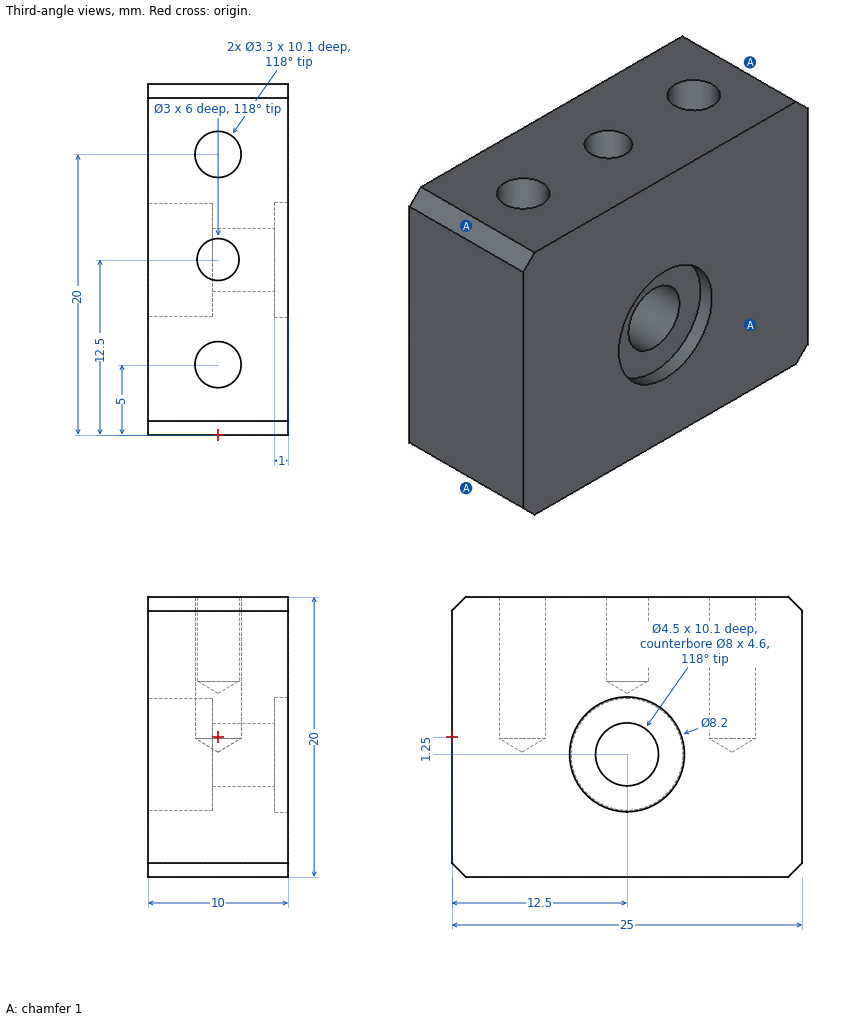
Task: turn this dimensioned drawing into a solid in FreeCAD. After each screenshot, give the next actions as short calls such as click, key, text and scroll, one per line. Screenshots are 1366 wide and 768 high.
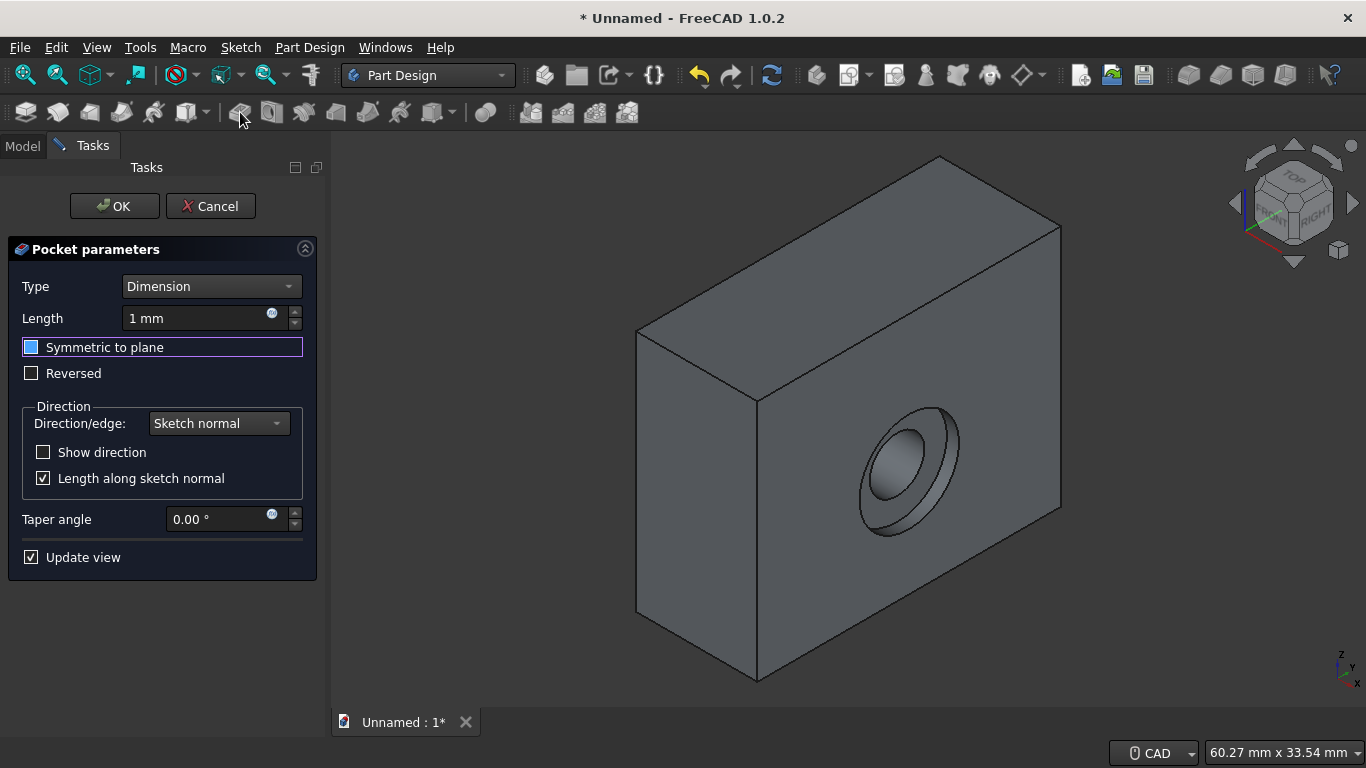
click(115, 206)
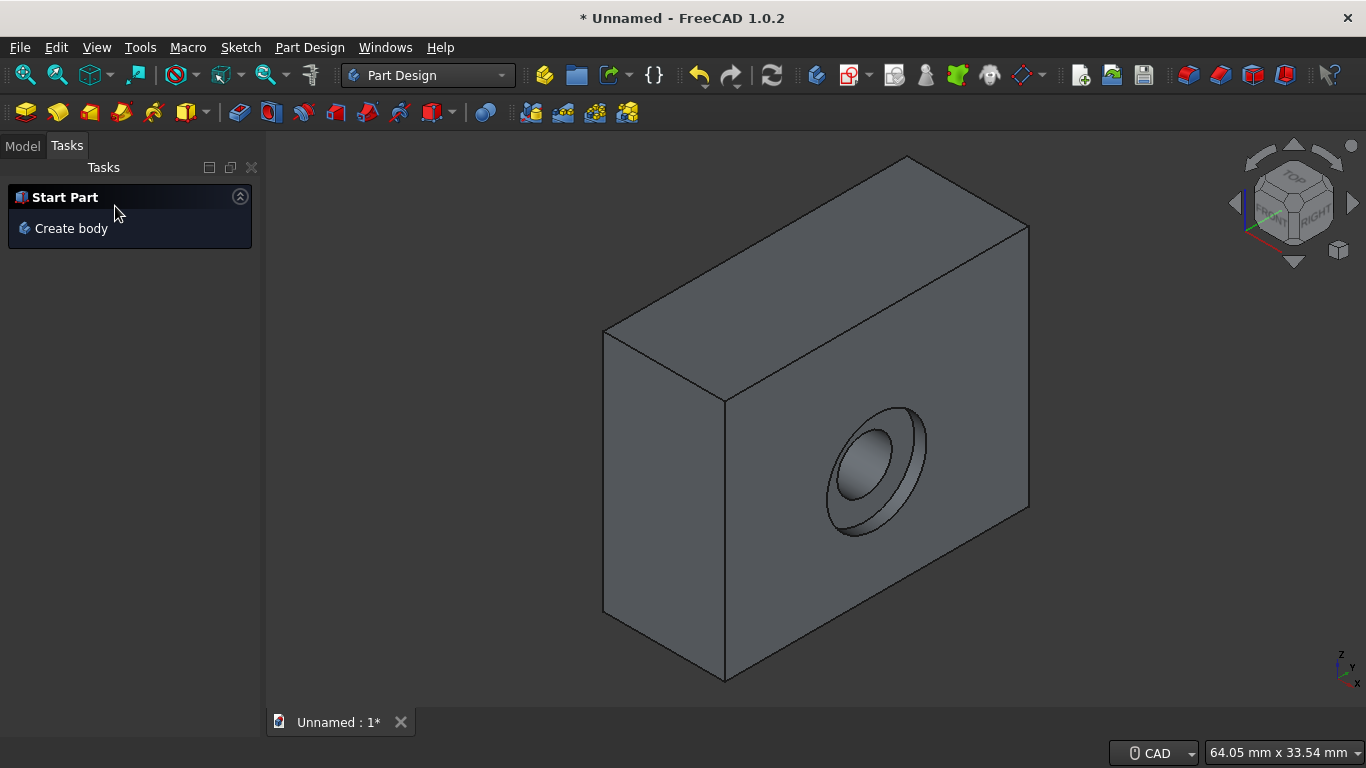
click(903, 228)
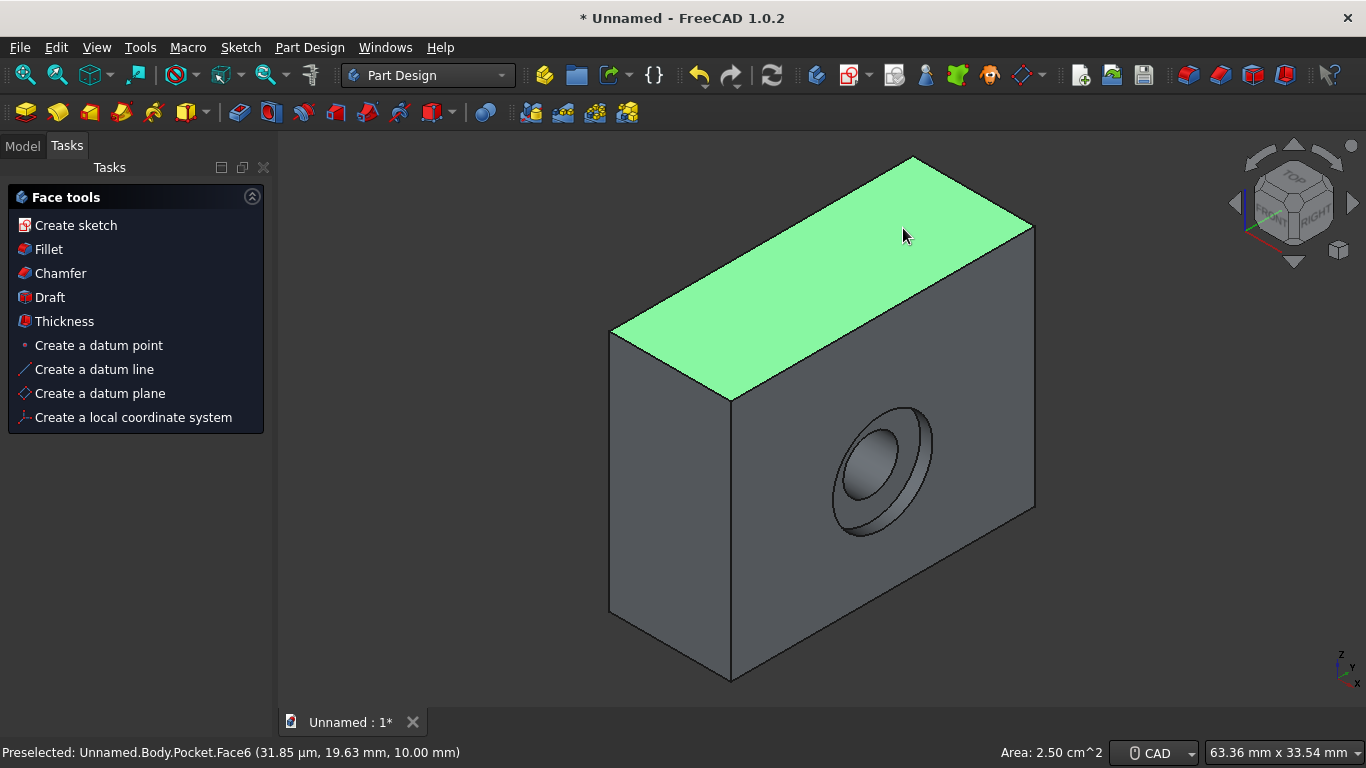
click(850, 76)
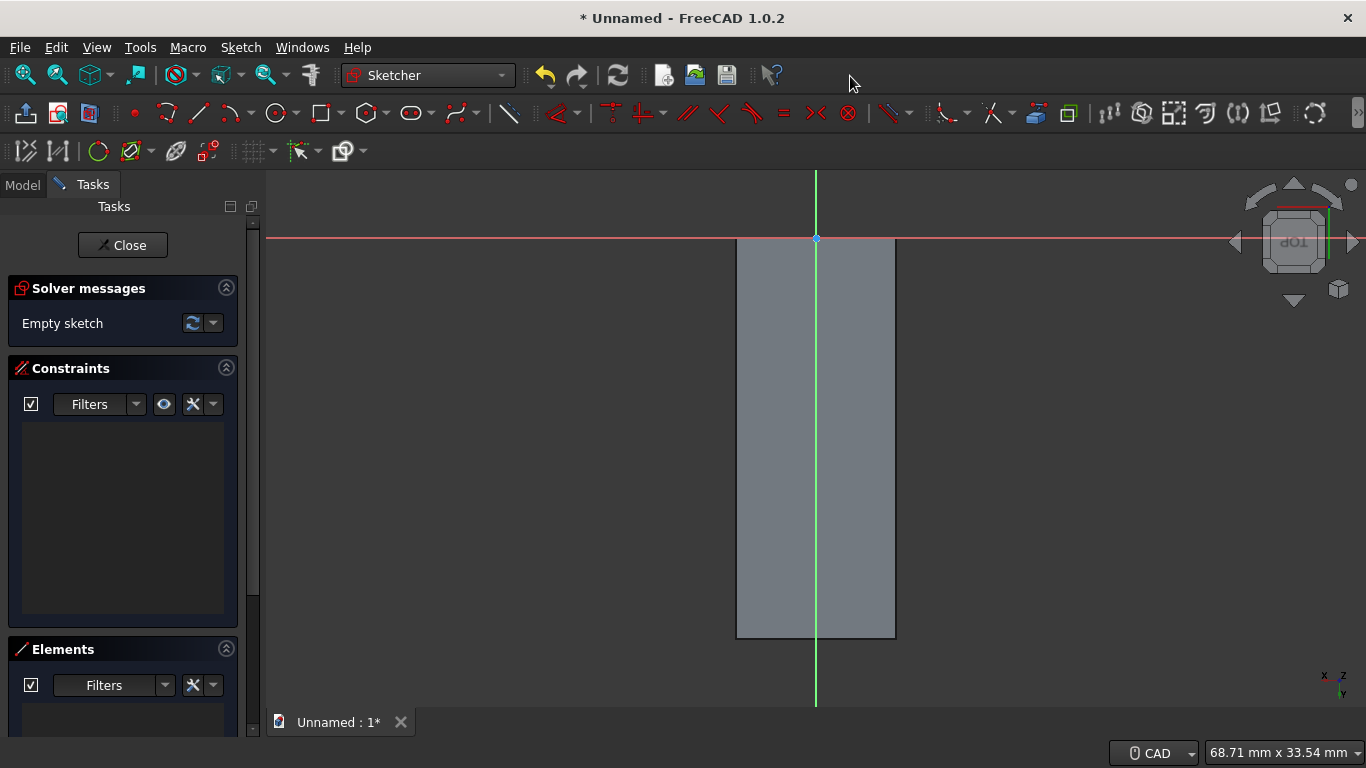
click(276, 114)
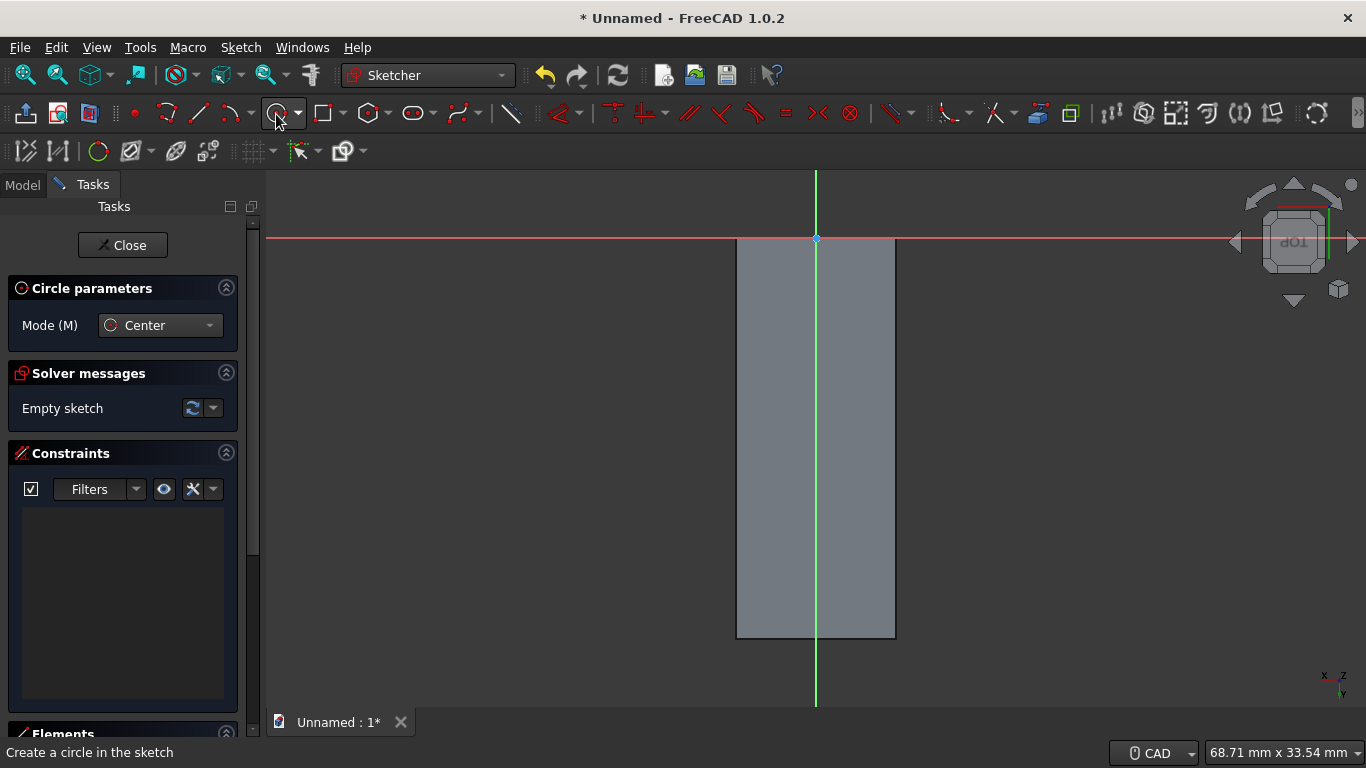
click(816, 559)
click(835, 540)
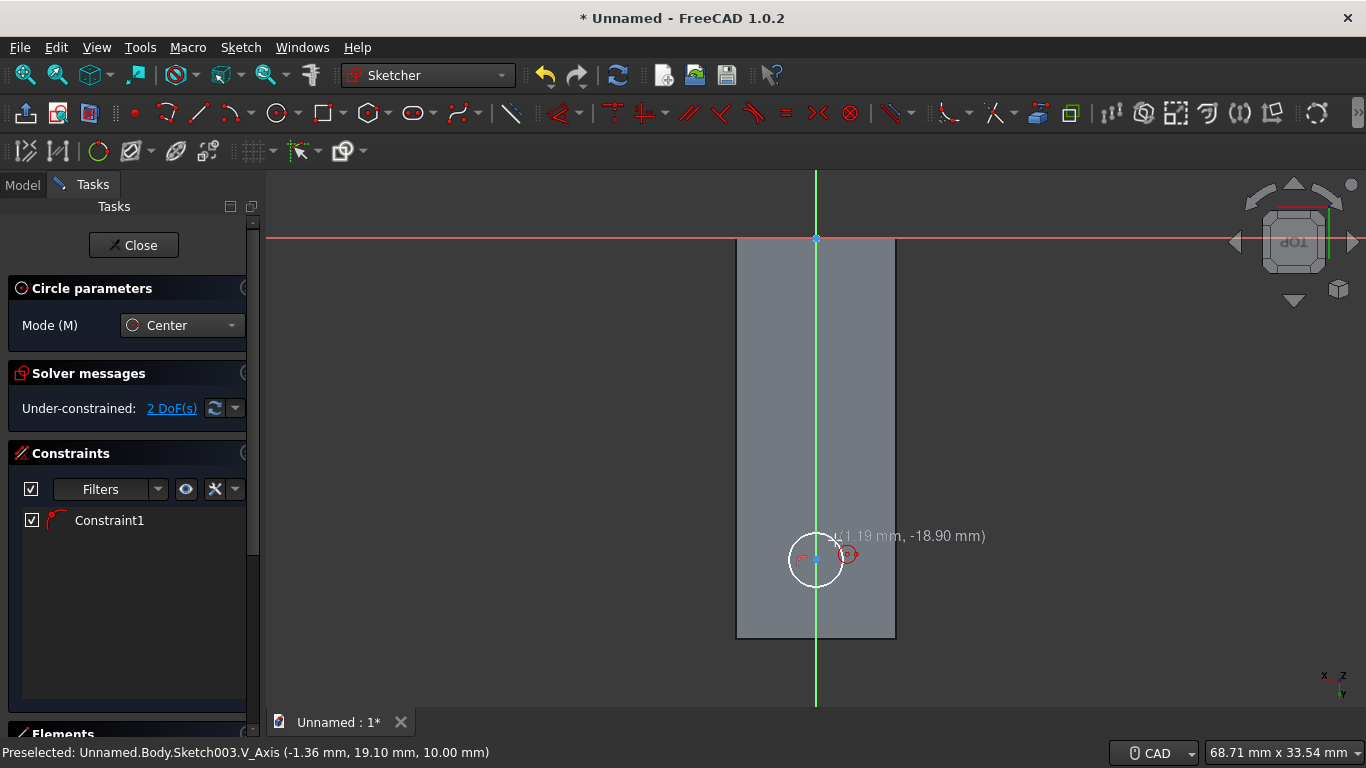
click(816, 318)
click(835, 300)
key(Escape)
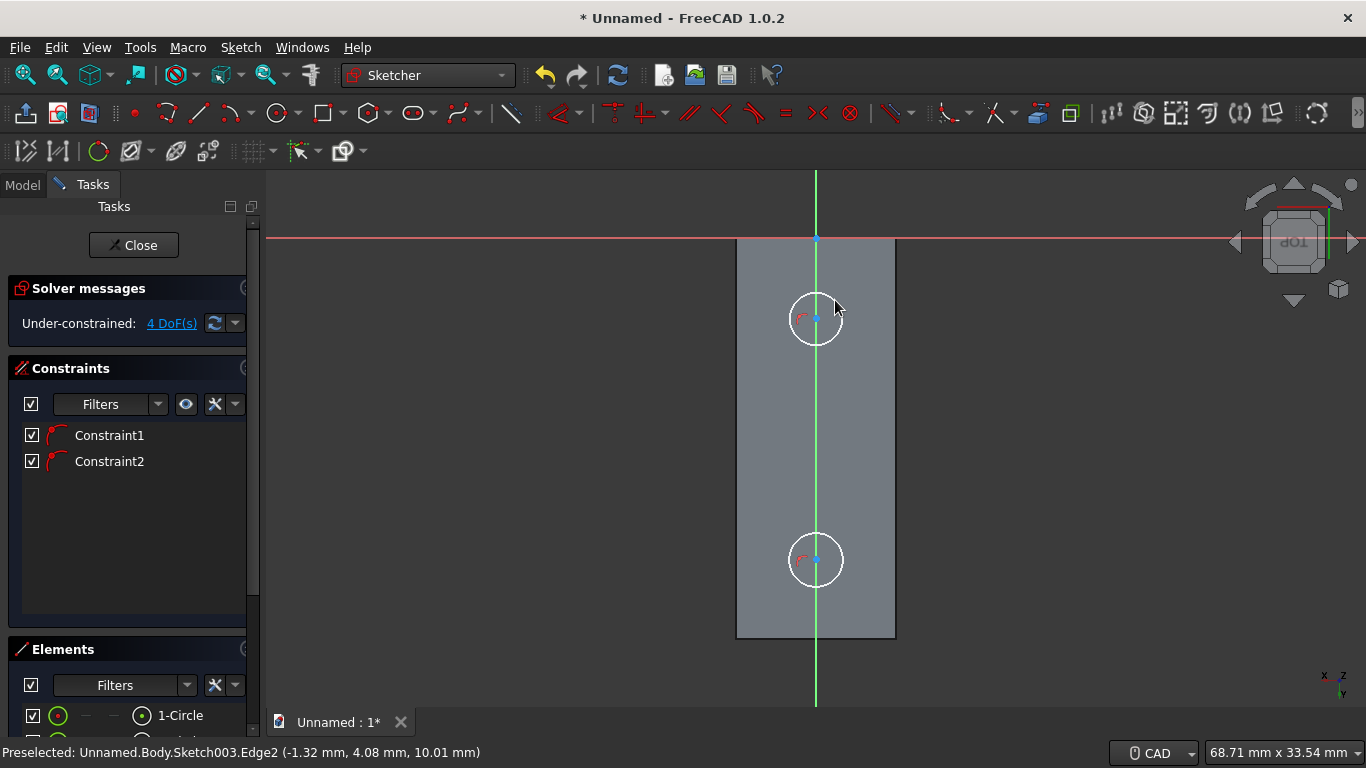
click(835, 541)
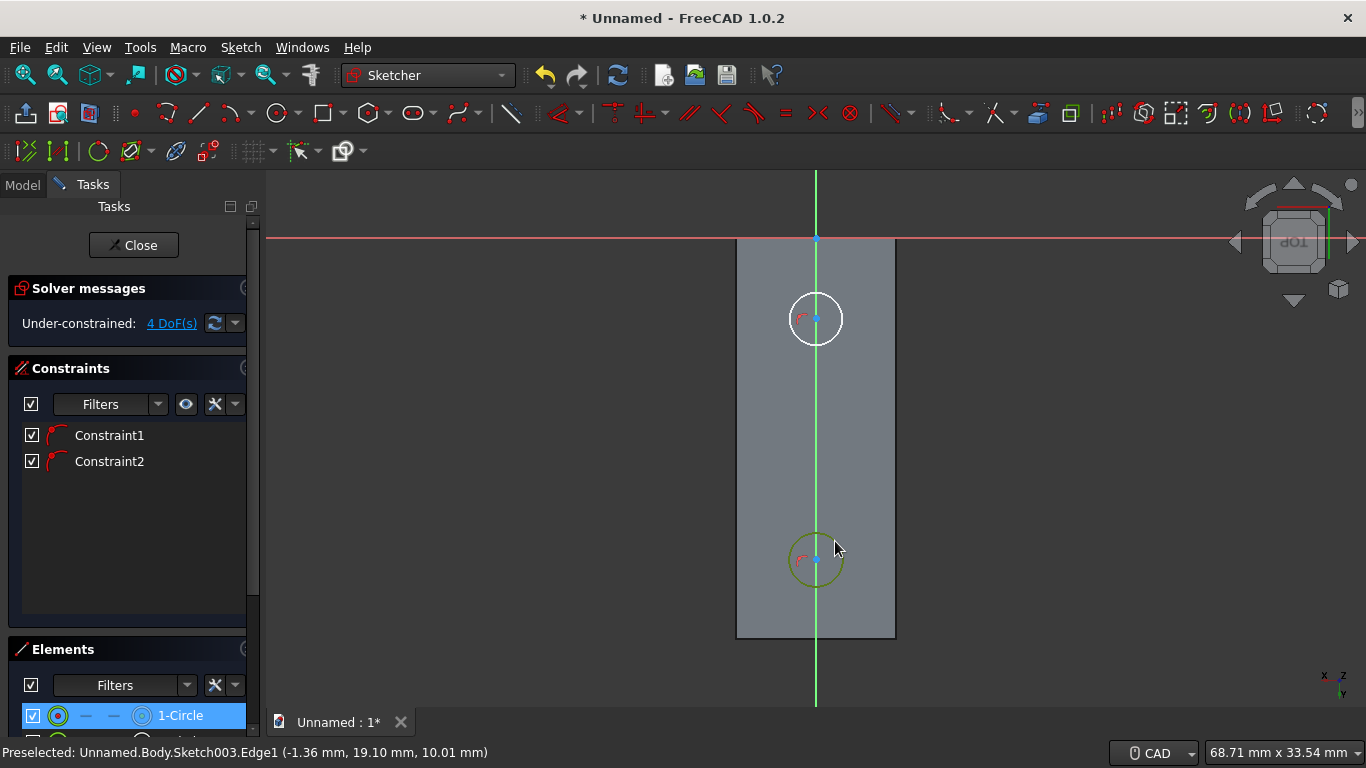
click(834, 300)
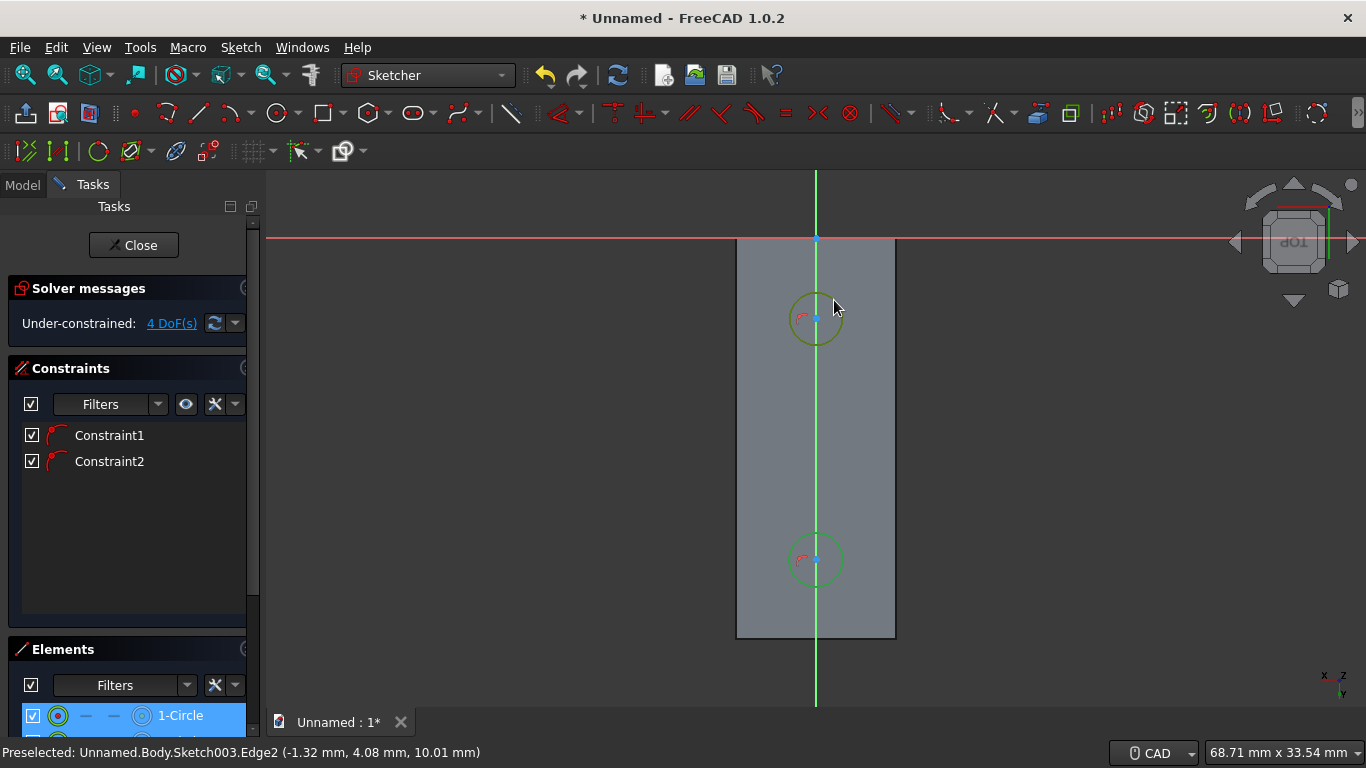
click(786, 114)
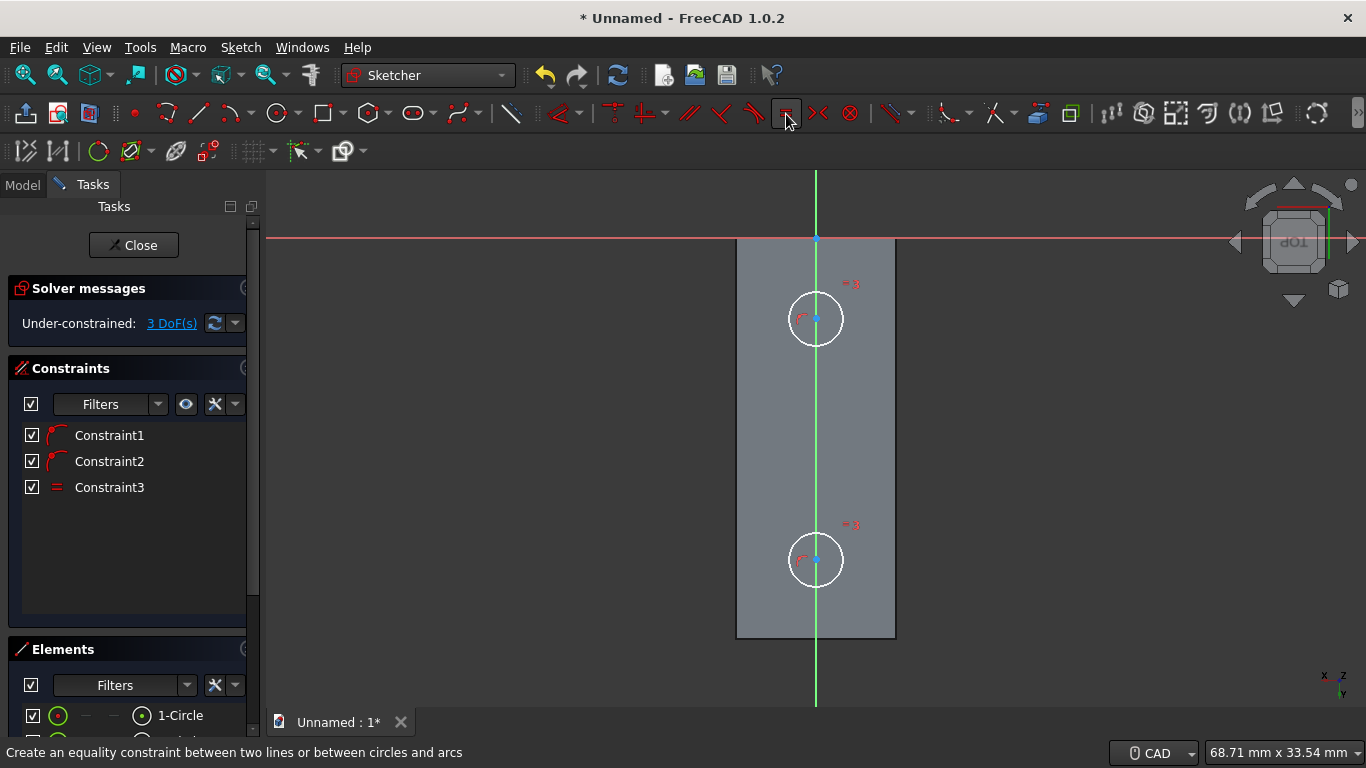
click(558, 114)